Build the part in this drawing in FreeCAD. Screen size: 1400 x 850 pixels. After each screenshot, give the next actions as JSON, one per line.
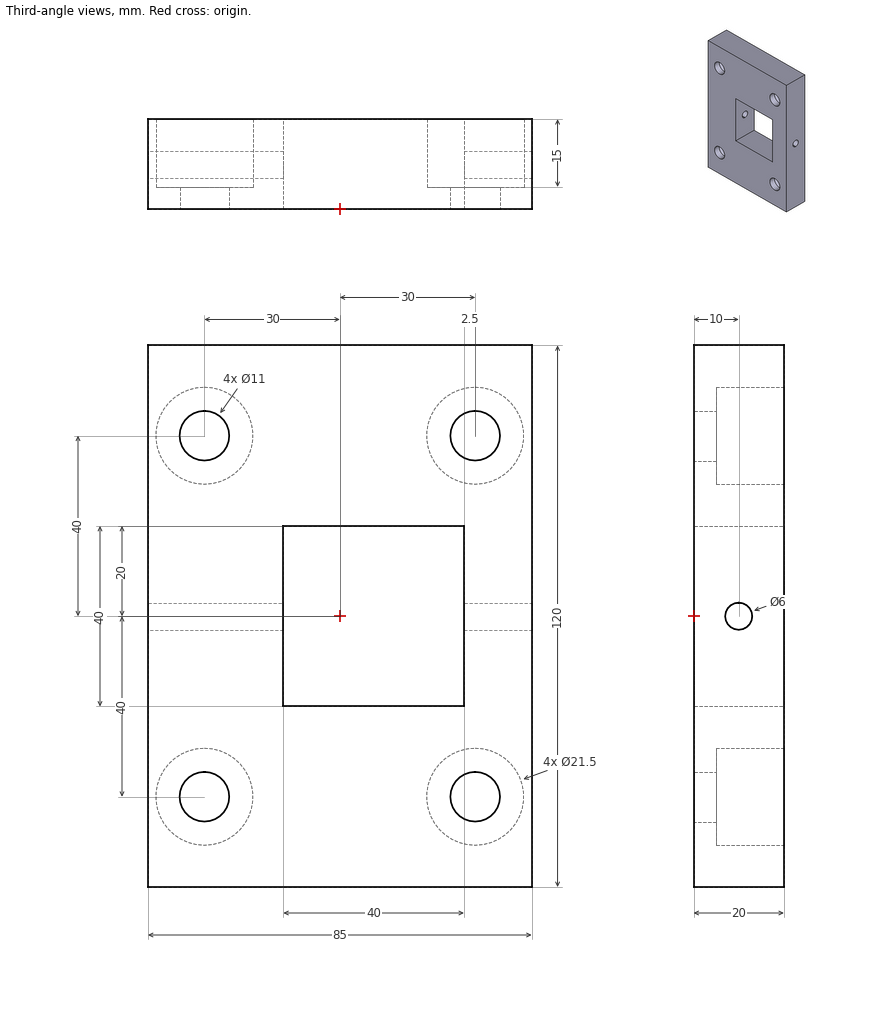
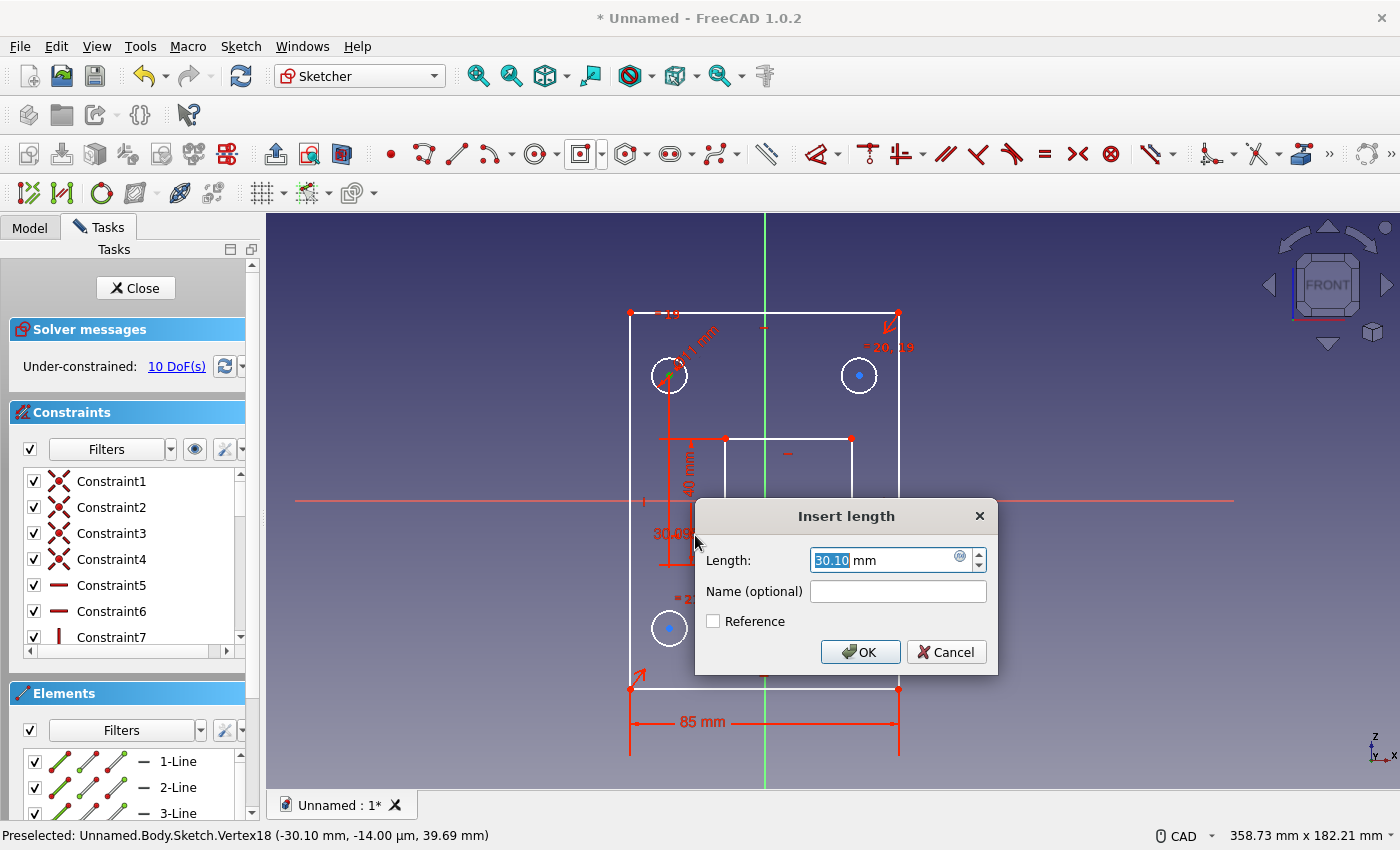
{"action": "type", "text": "30"}
{"action": "key", "text": "Return"}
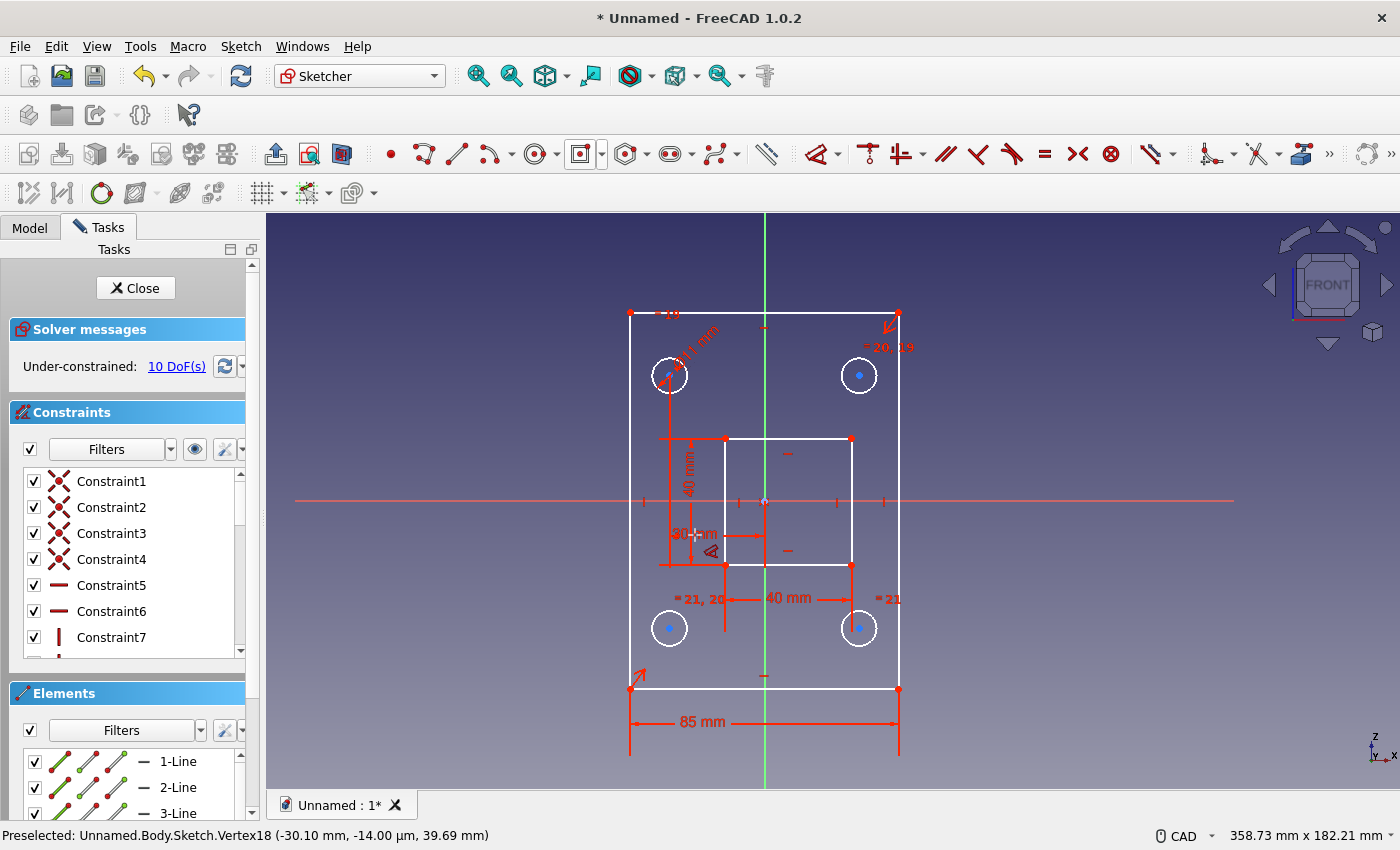
{"action": "left_click", "coordinate": [670, 376]}
{"action": "left_click", "coordinate": [799, 410]}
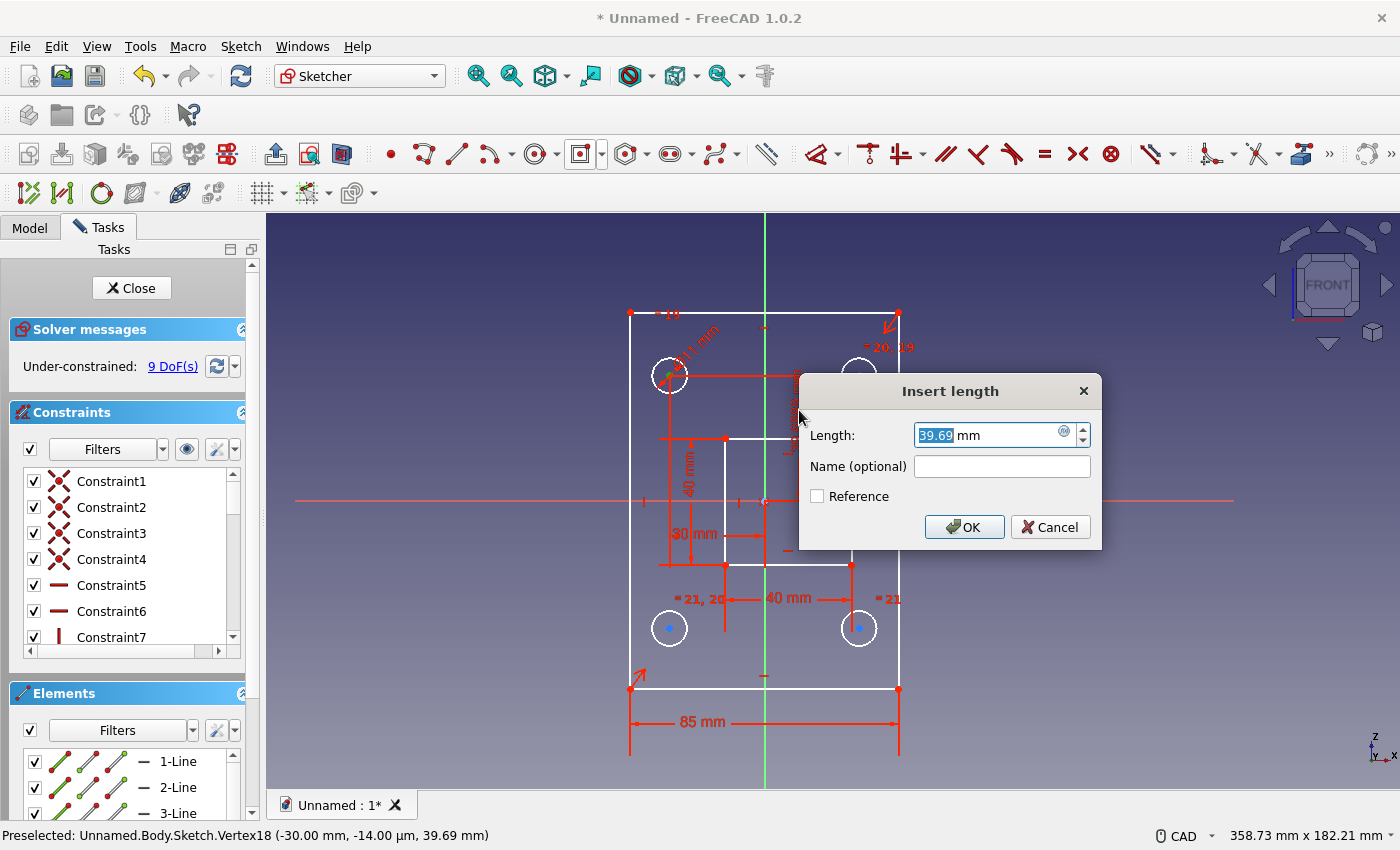
{"action": "type", "text": "40"}
{"action": "key", "text": "Return"}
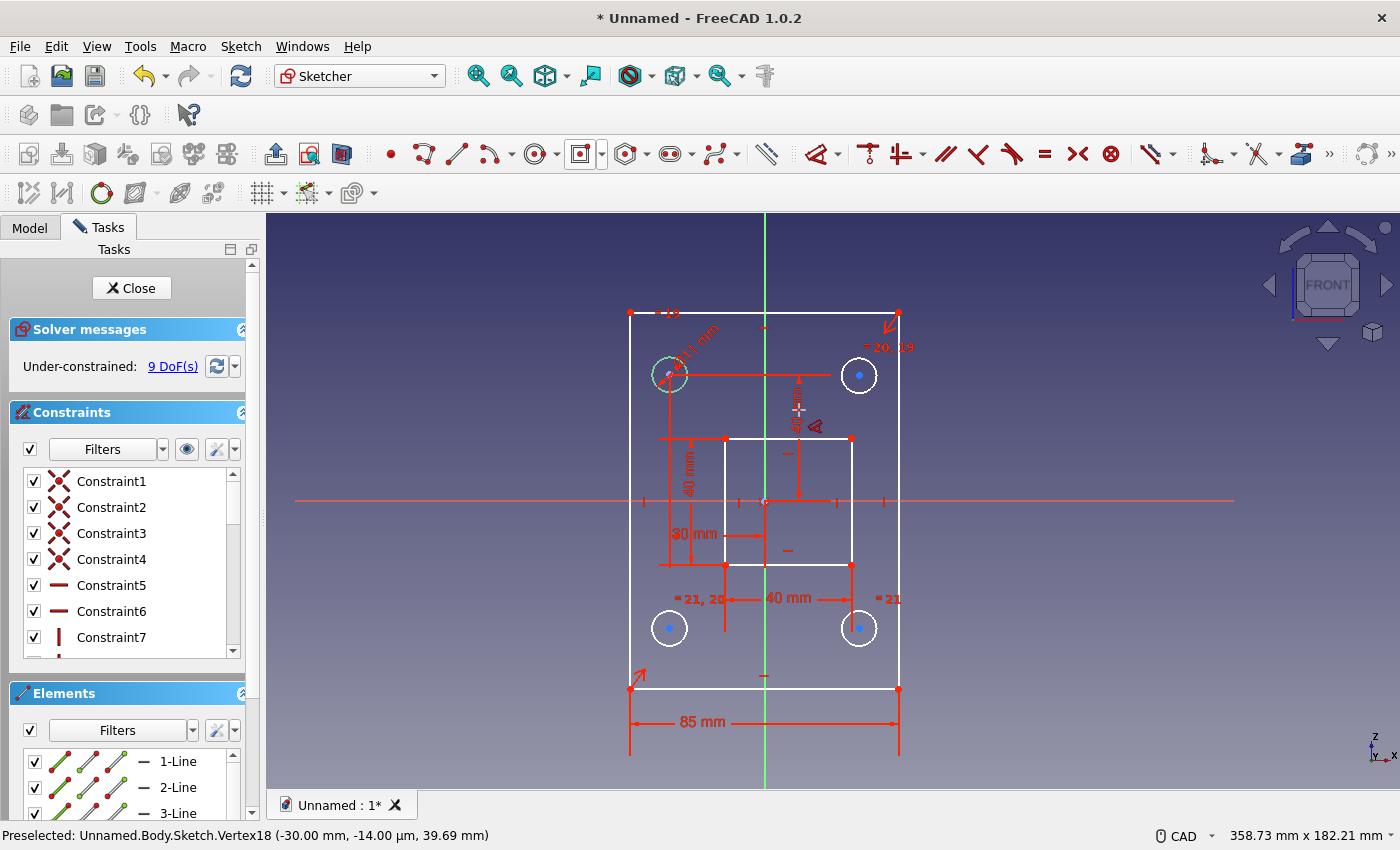
{"action": "left_click", "coordinate": [859, 376]}
{"action": "left_click", "coordinate": [812, 342]}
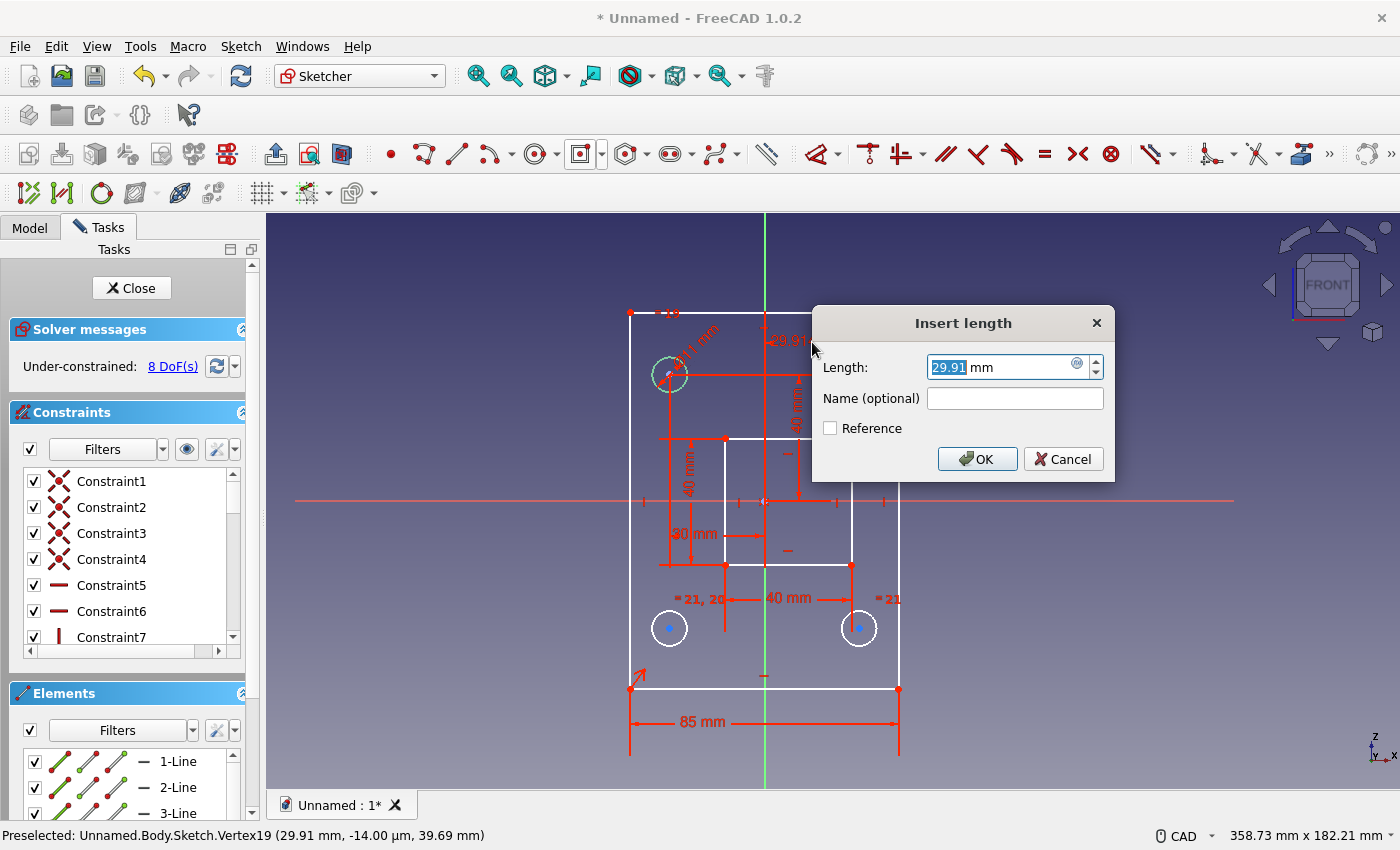
{"action": "type", "text": "30"}
{"action": "key", "text": "Return"}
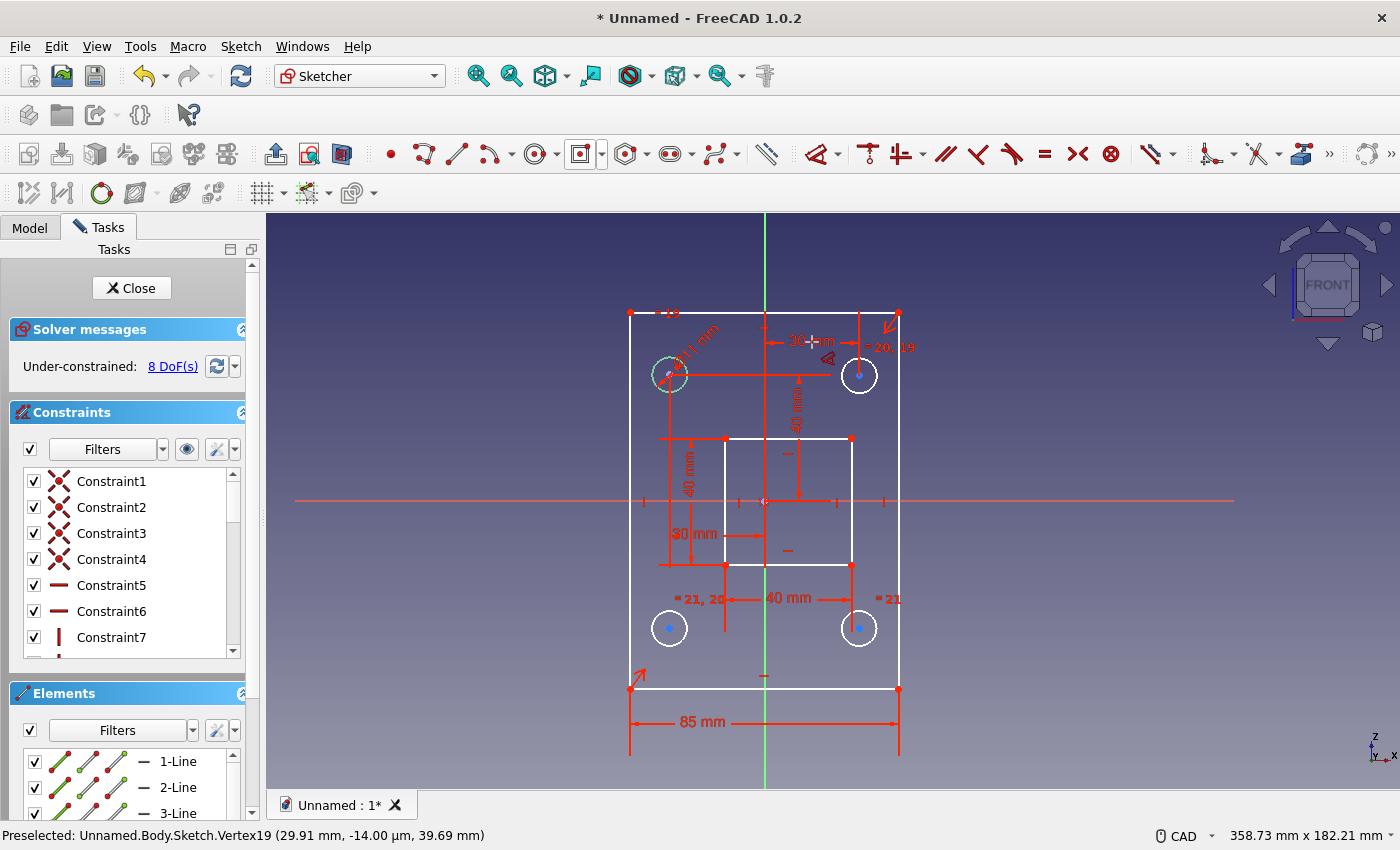
{"action": "left_click", "coordinate": [859, 376]}
{"action": "left_click", "coordinate": [917, 438]}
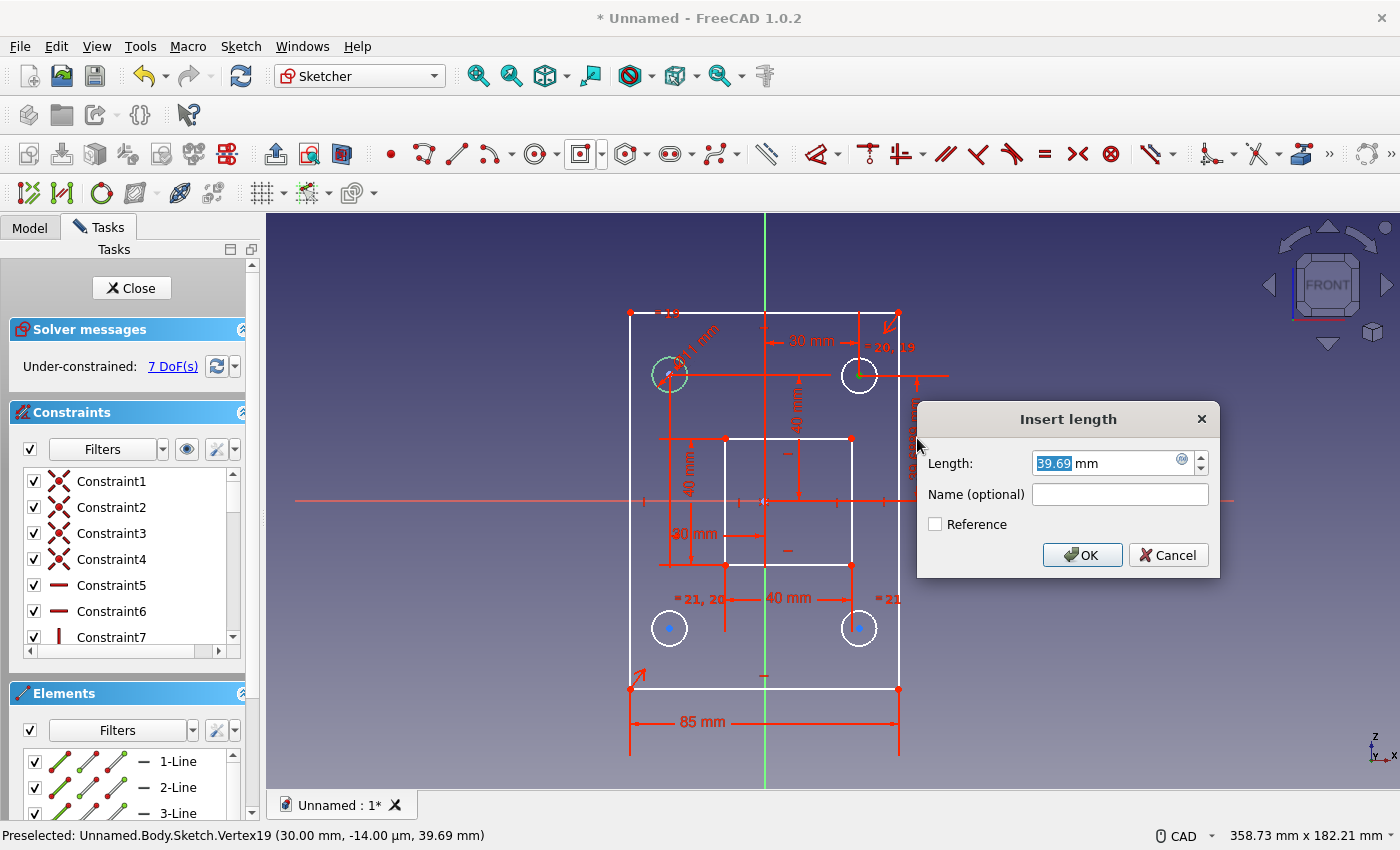
{"action": "type", "text": "40"}
{"action": "key", "text": "Return"}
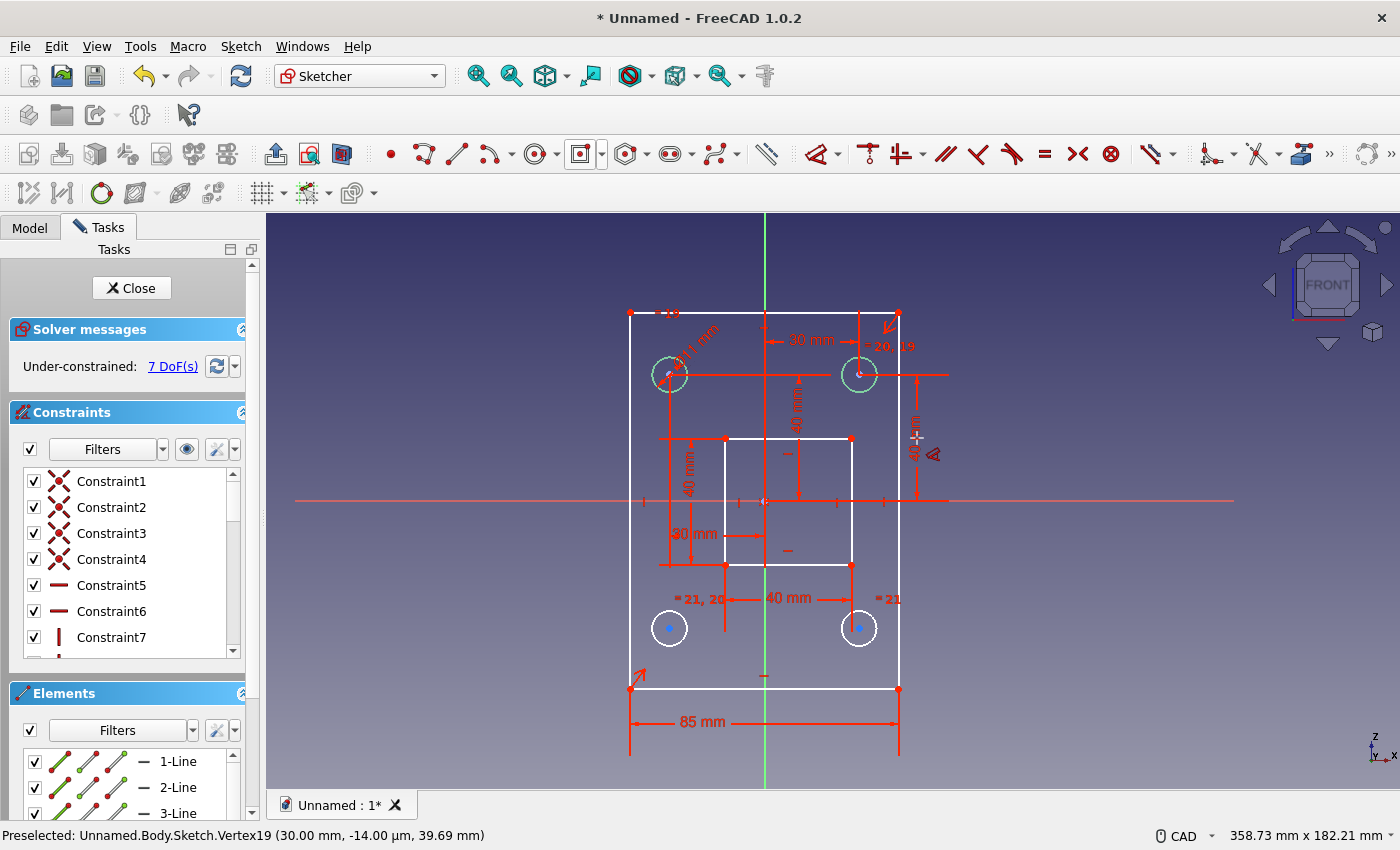
{"action": "left_click", "coordinate": [669, 628]}
{"action": "left_click", "coordinate": [717, 662]}